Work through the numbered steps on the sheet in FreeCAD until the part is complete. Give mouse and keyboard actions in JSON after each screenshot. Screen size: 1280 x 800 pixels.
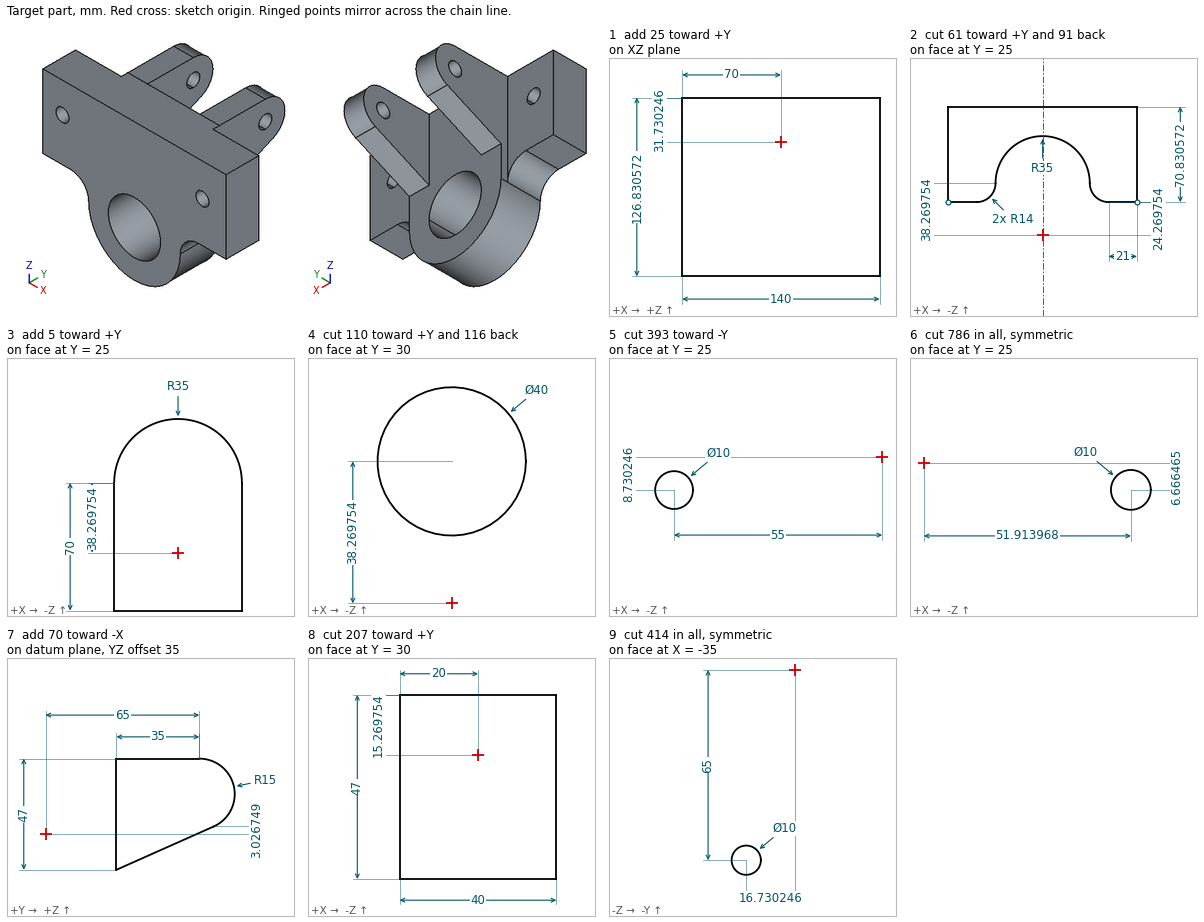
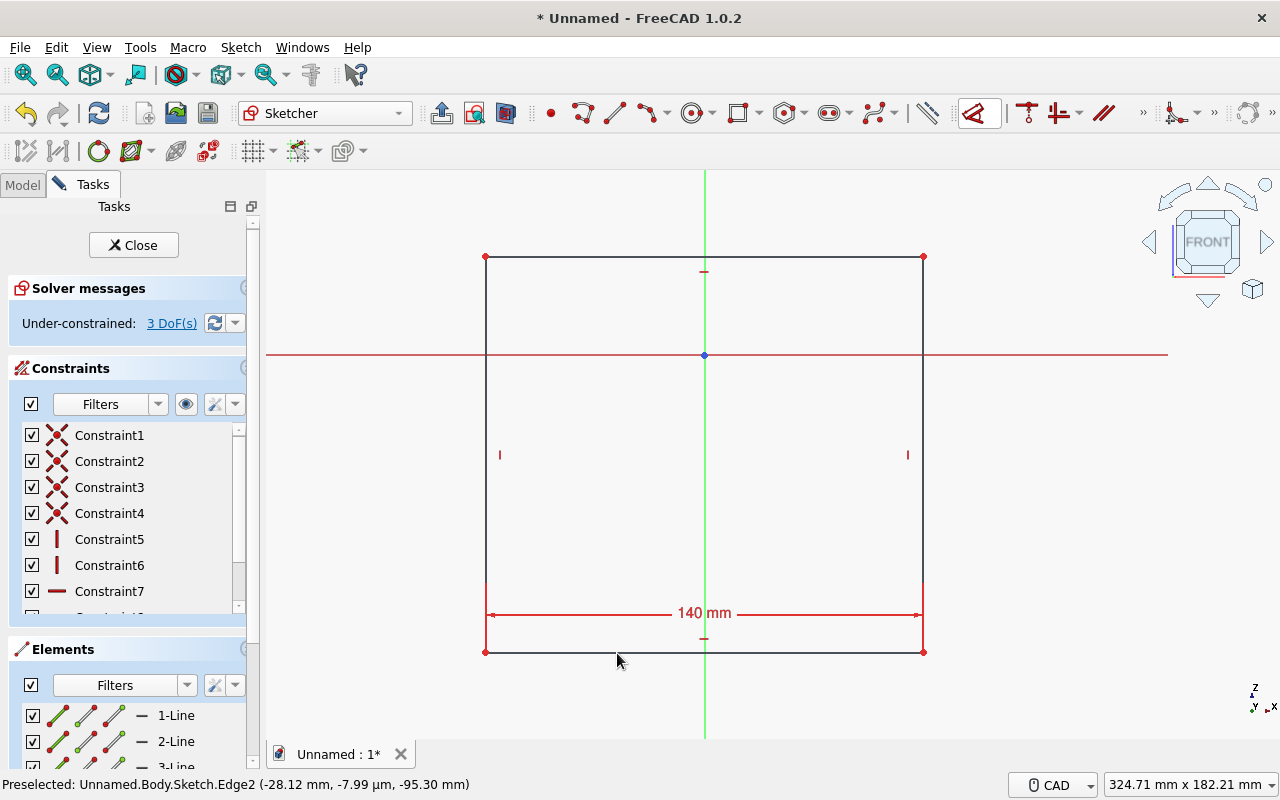
{"action": "left_click", "coordinate": [486, 257]}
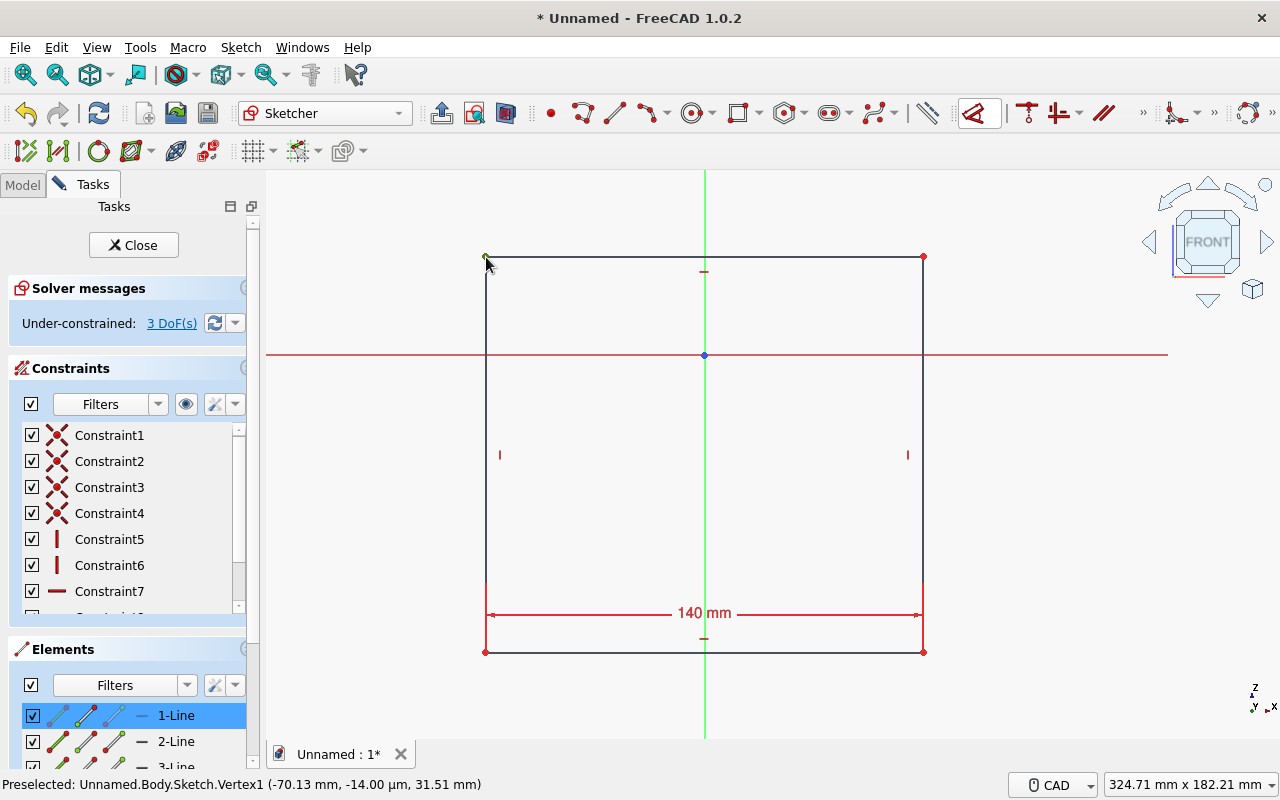
{"action": "key", "text": "l"}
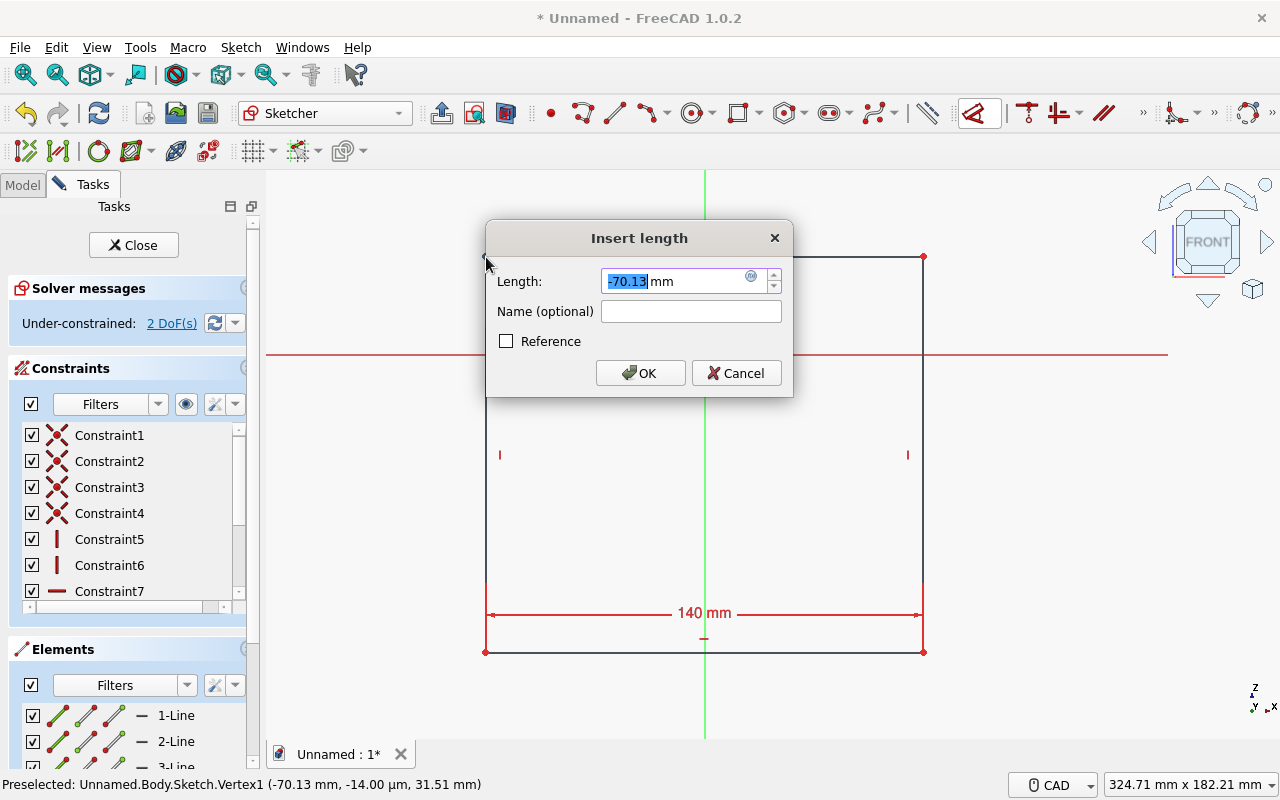
{"action": "type", "text": "-70"}
{"action": "key", "text": "Return"}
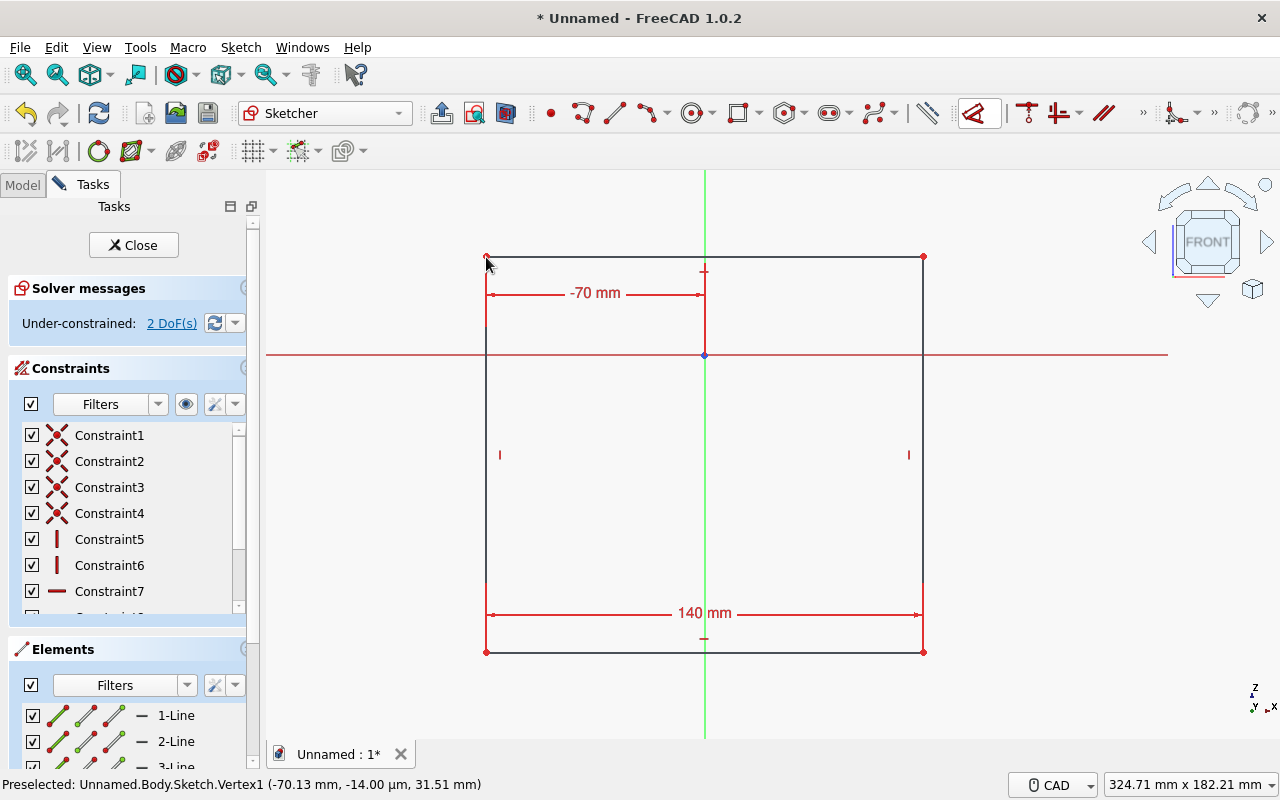
{"action": "left_click", "coordinate": [486, 376]}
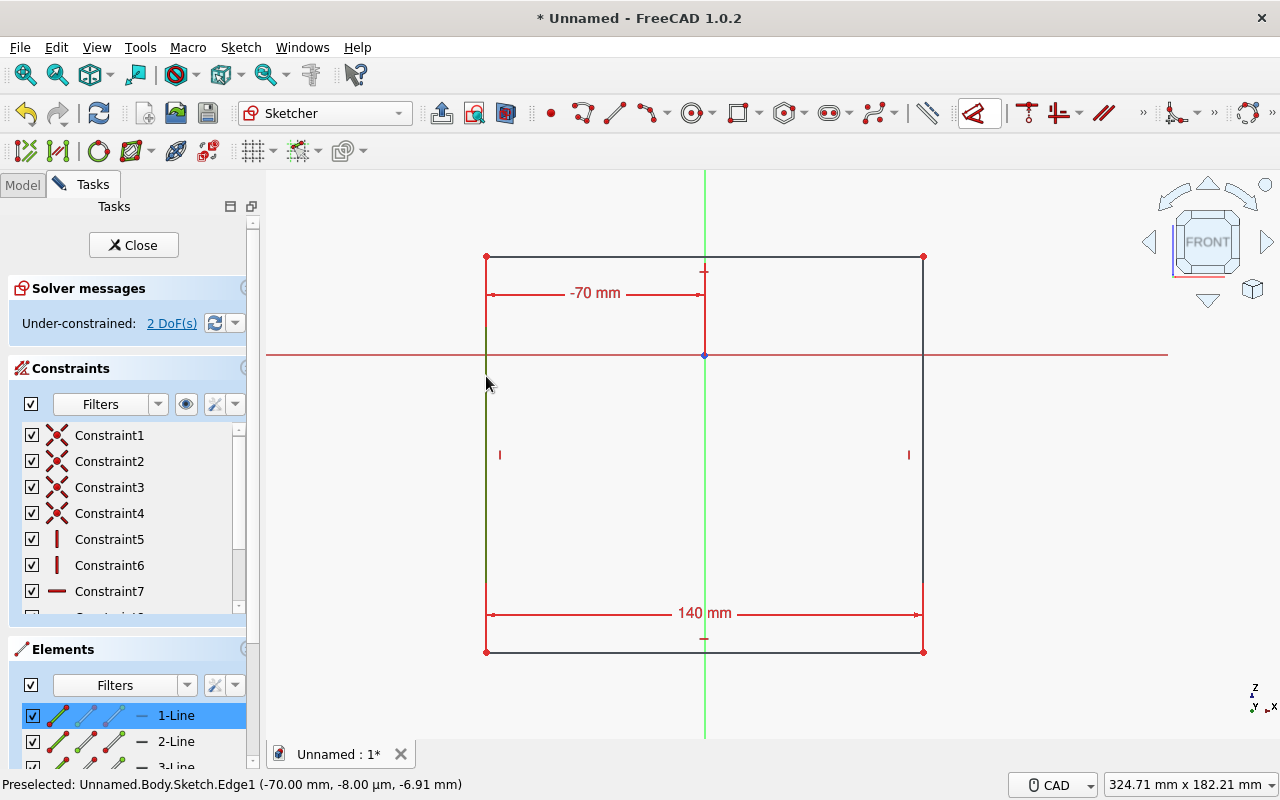
{"action": "key", "text": "i"}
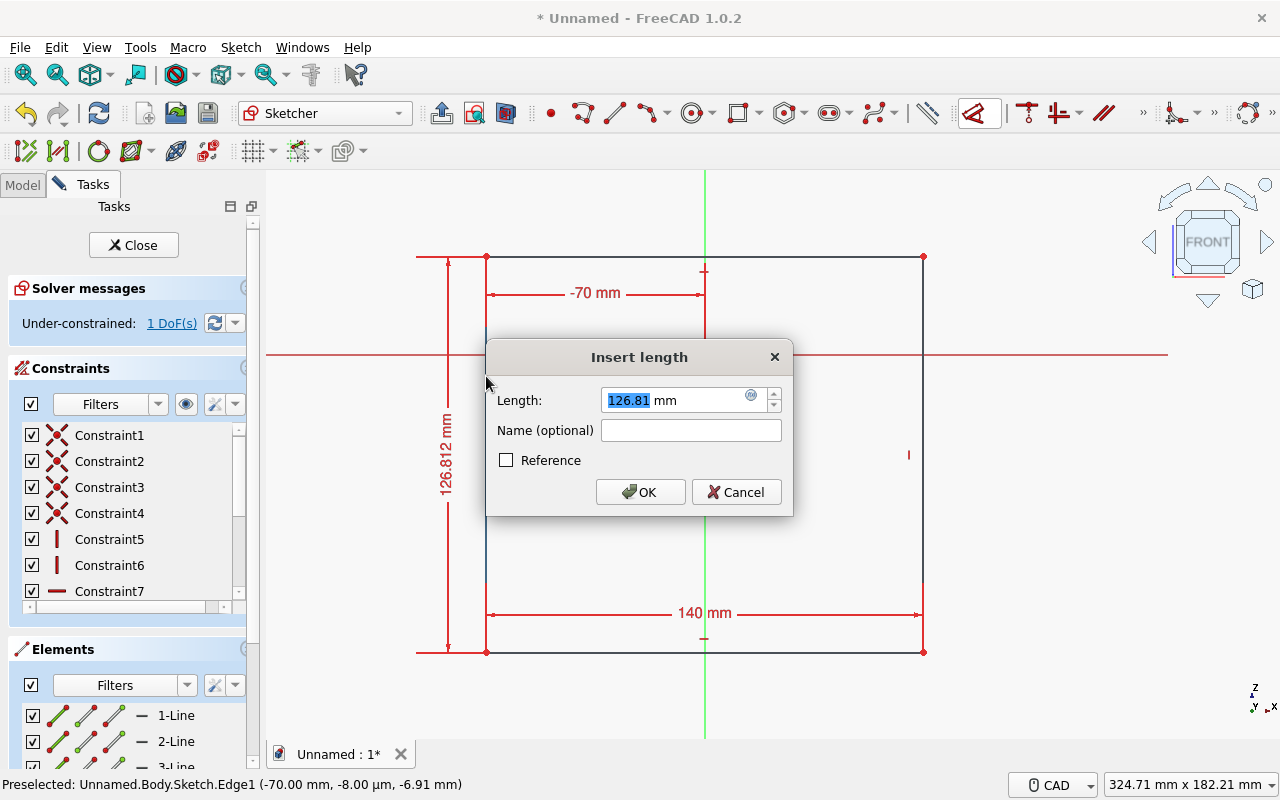
{"action": "type", "text": "126.830572"}
{"action": "key", "text": "Return"}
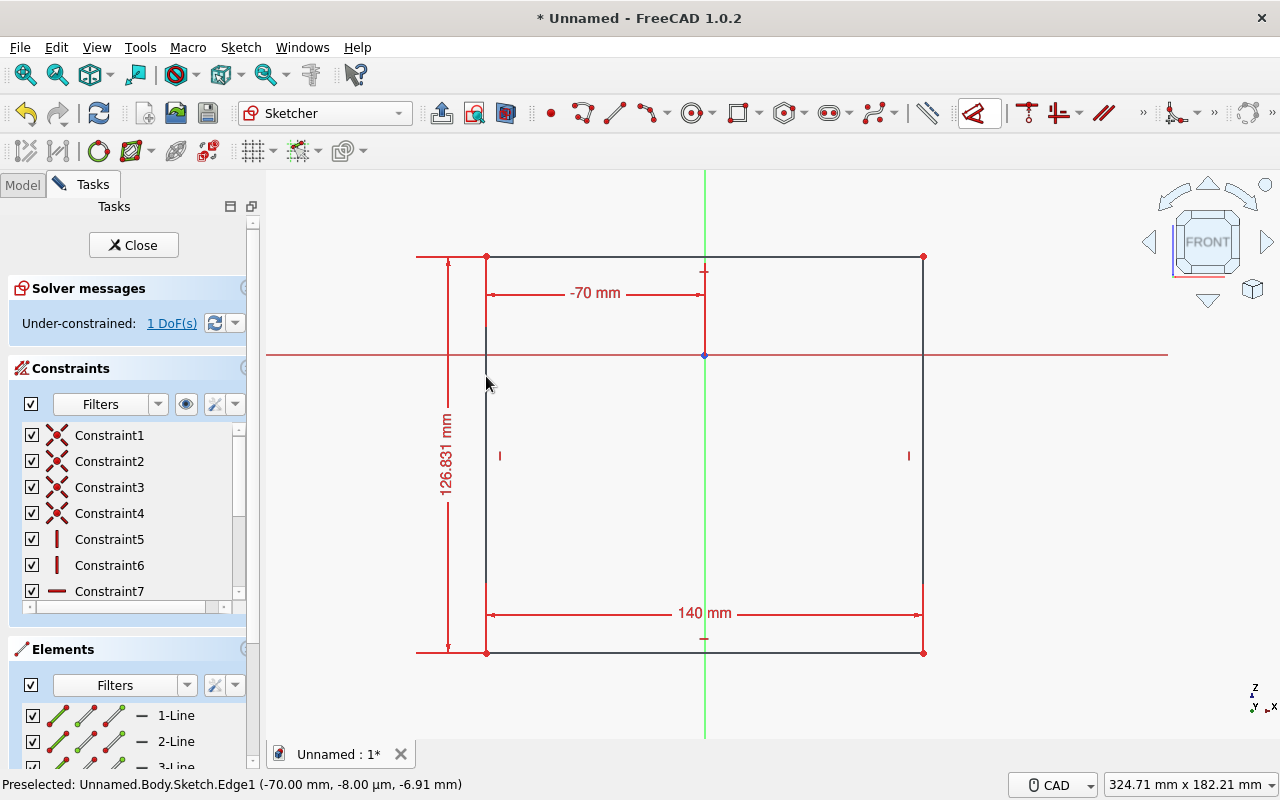
{"action": "left_click", "coordinate": [486, 257]}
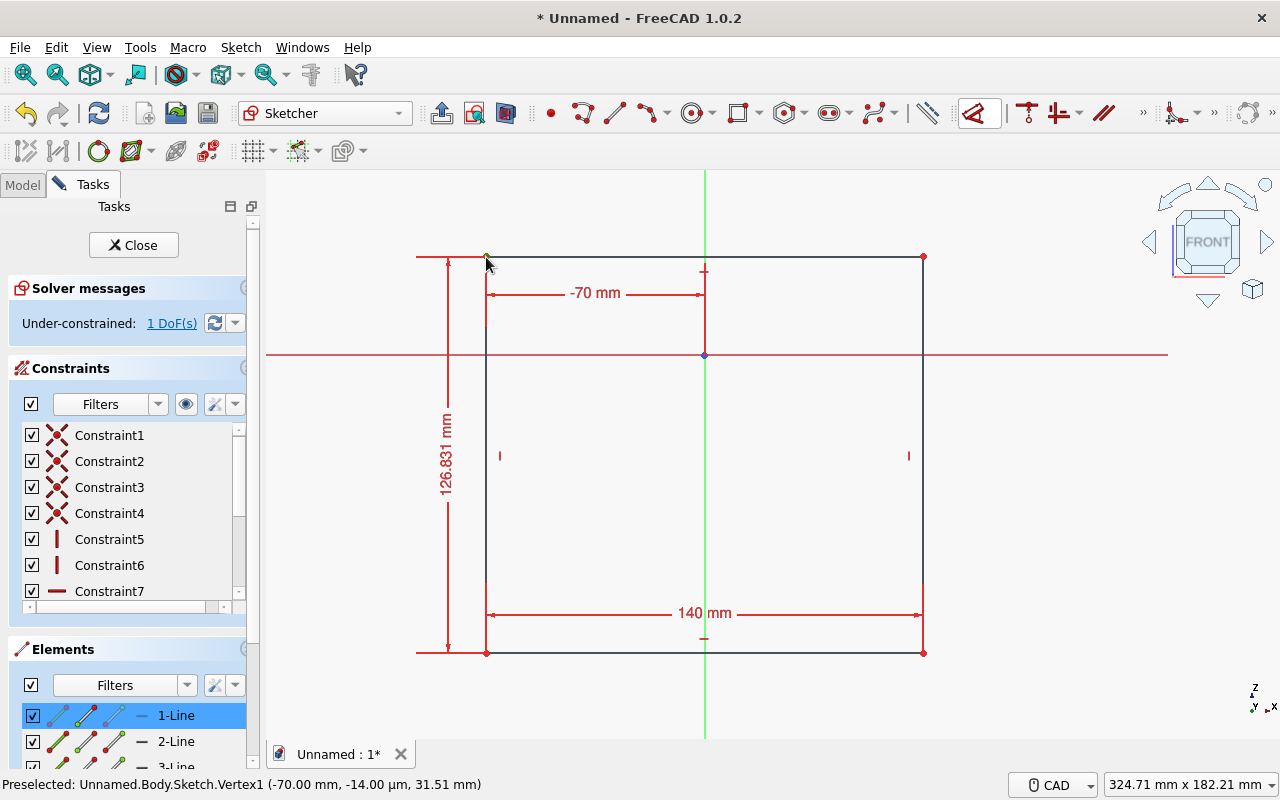
{"action": "key", "text": "i"}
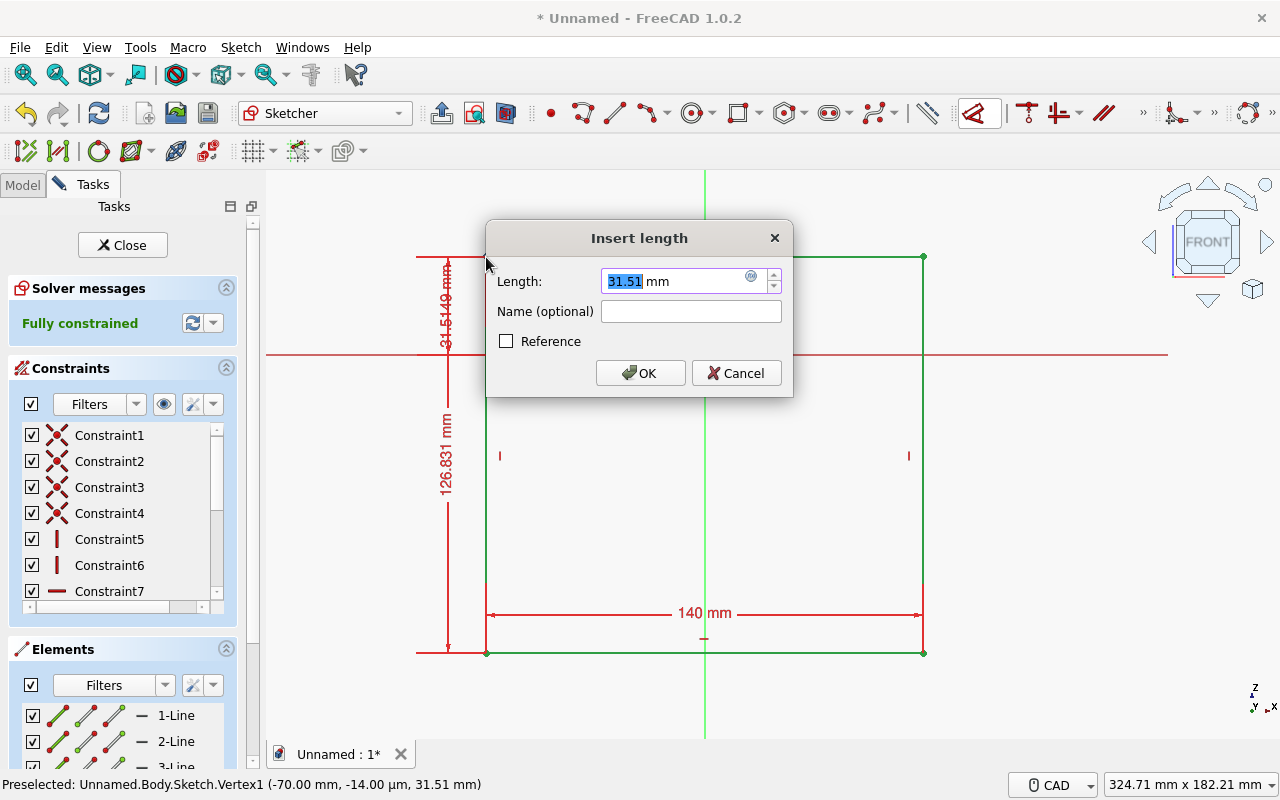
{"action": "type", "text": "31.730246"}
{"action": "key", "text": "Return"}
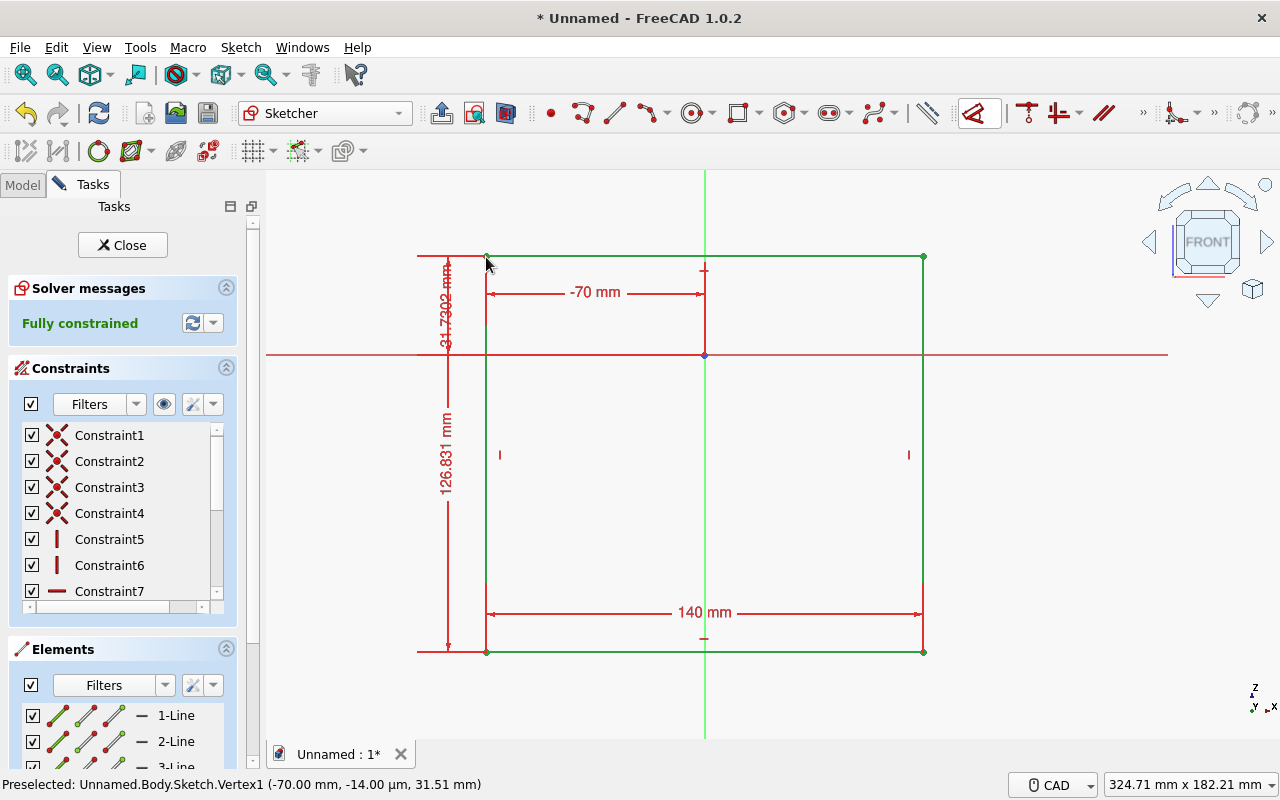
{"action": "left_click", "coordinate": [123, 245]}